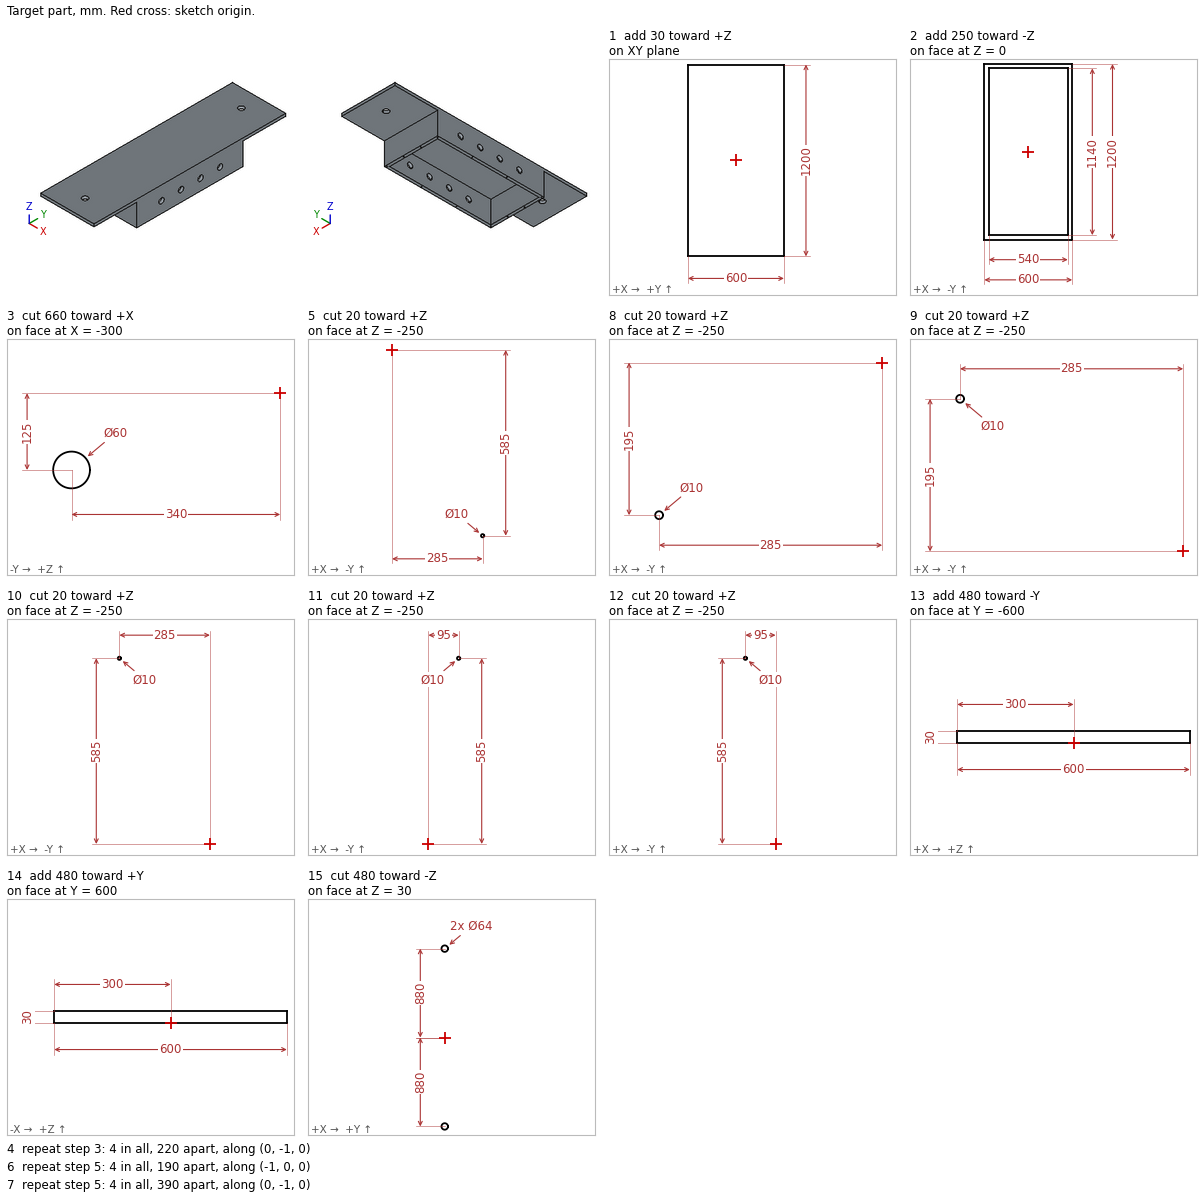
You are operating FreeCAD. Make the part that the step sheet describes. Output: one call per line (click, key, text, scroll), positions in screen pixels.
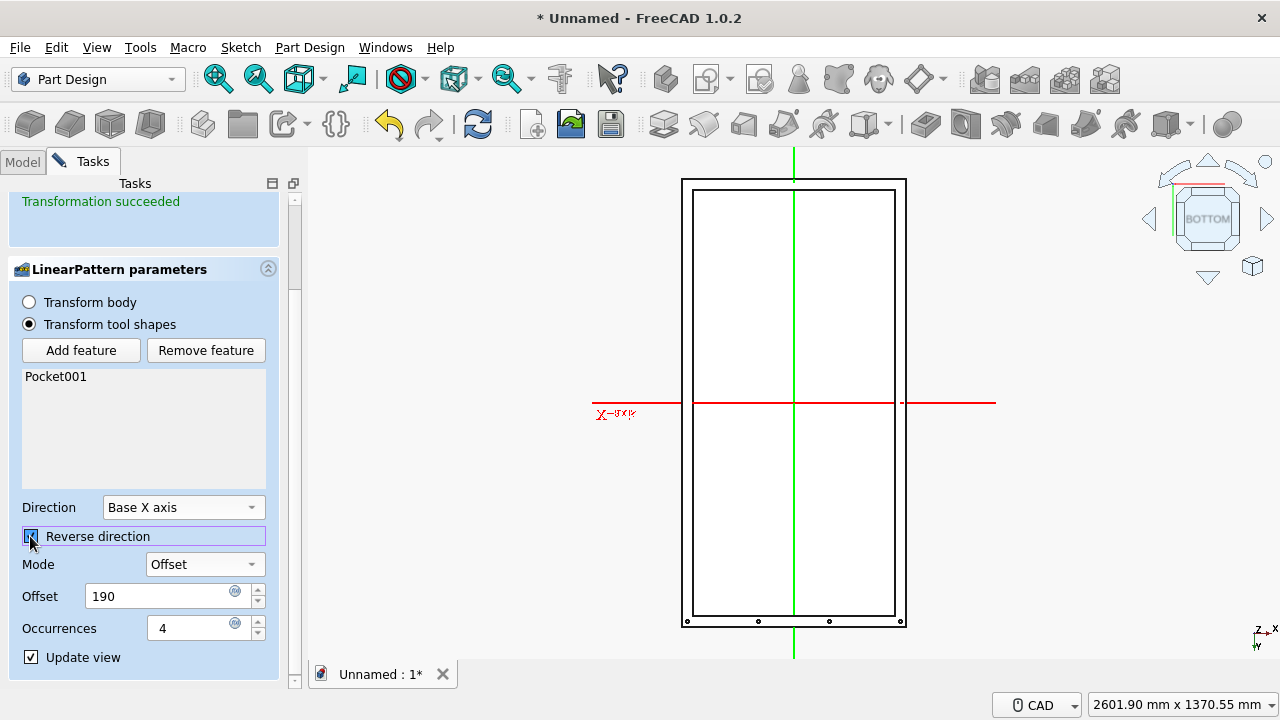
scroll(295, 440, up, 3)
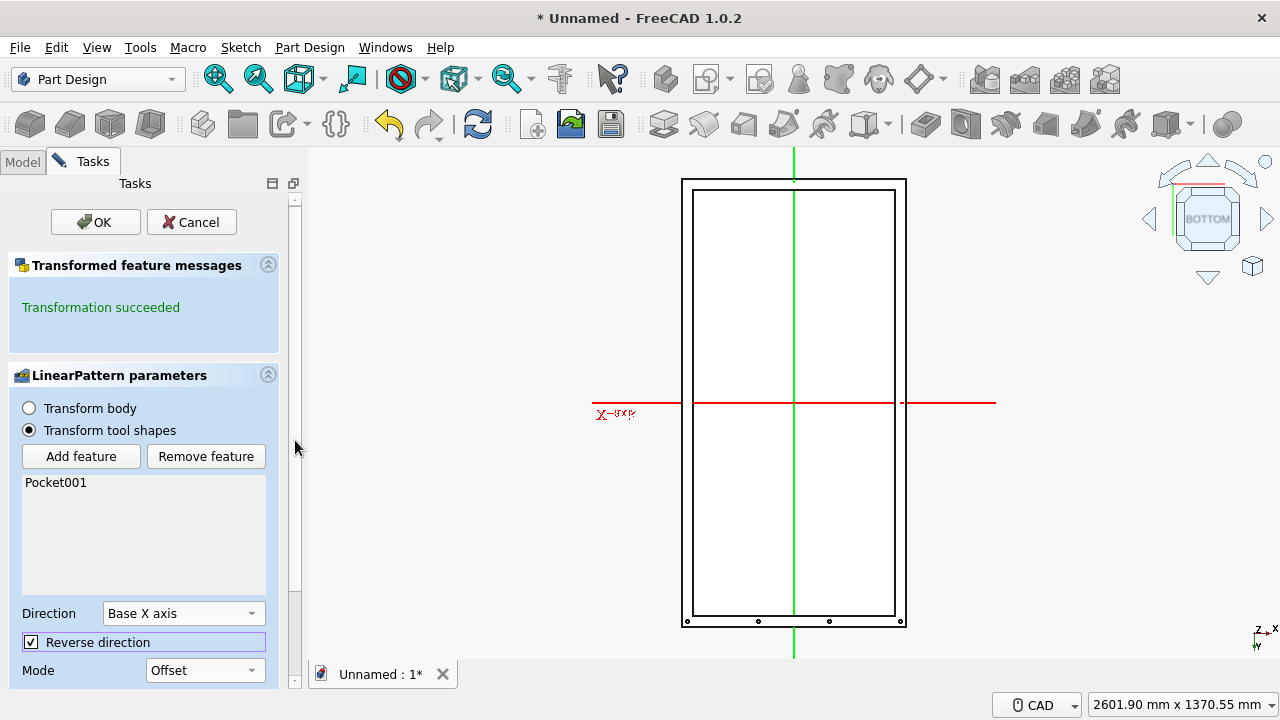
click(96, 222)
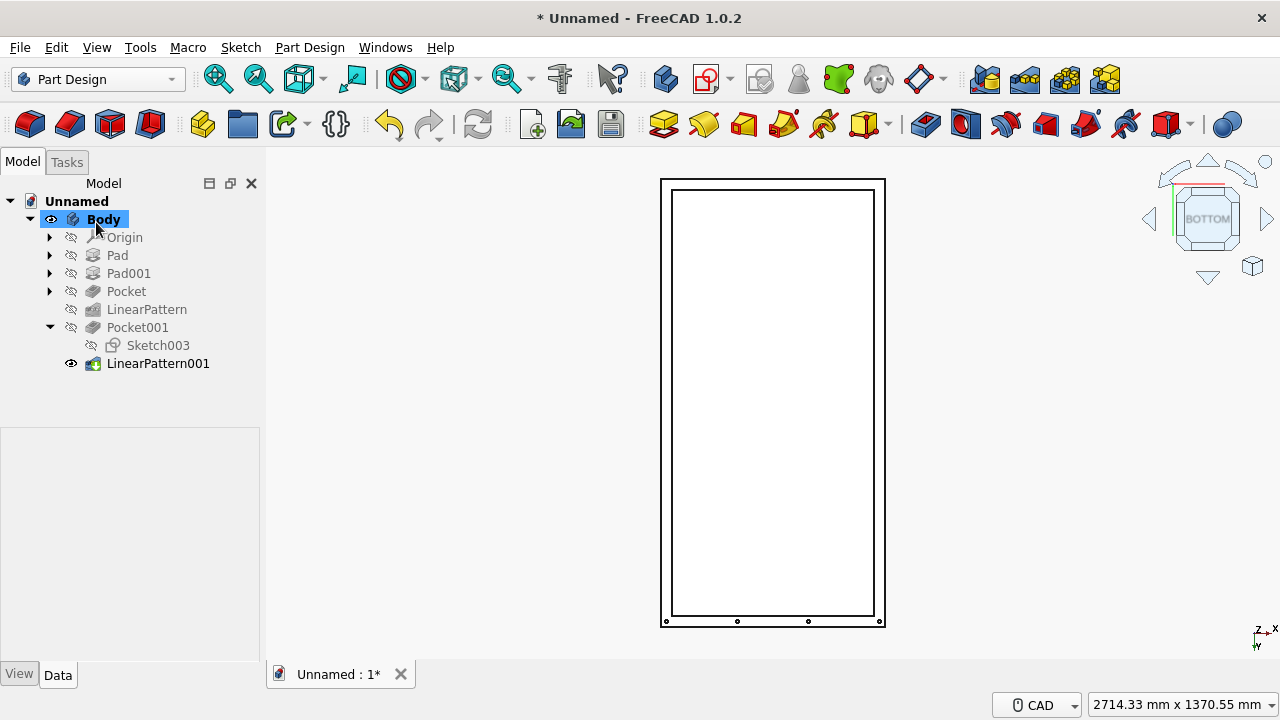
click(116, 327)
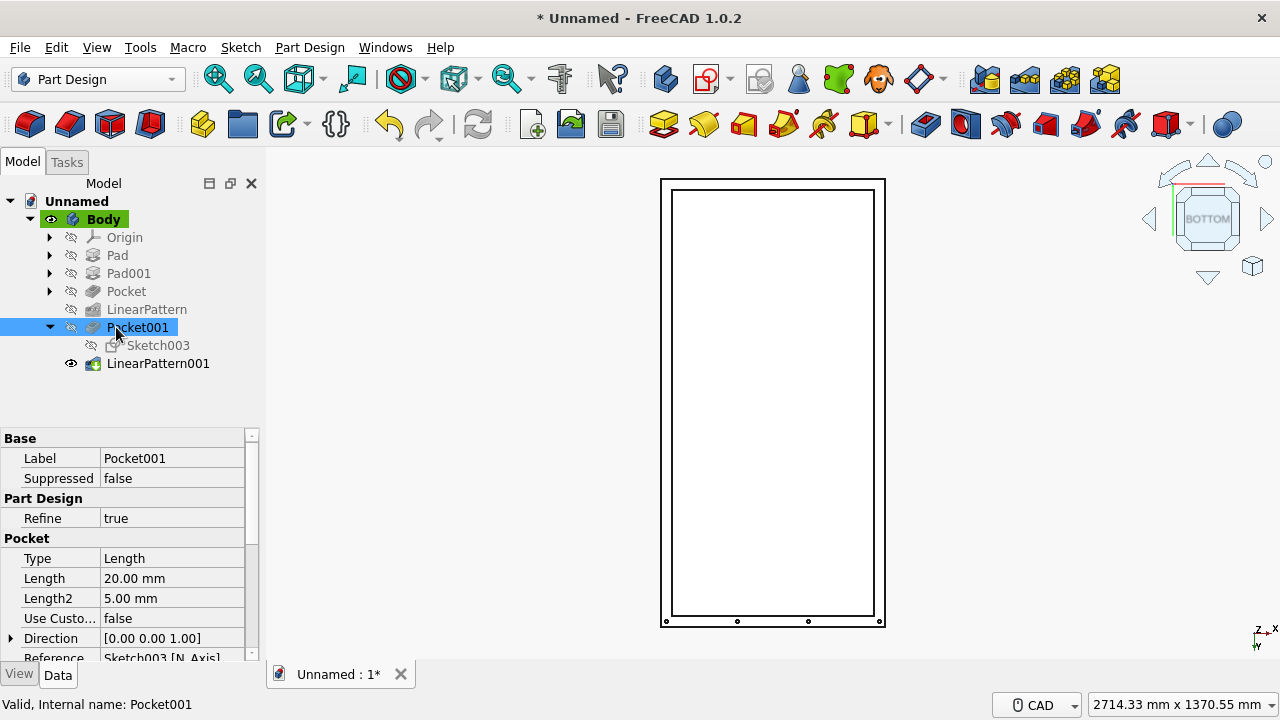
click(1026, 80)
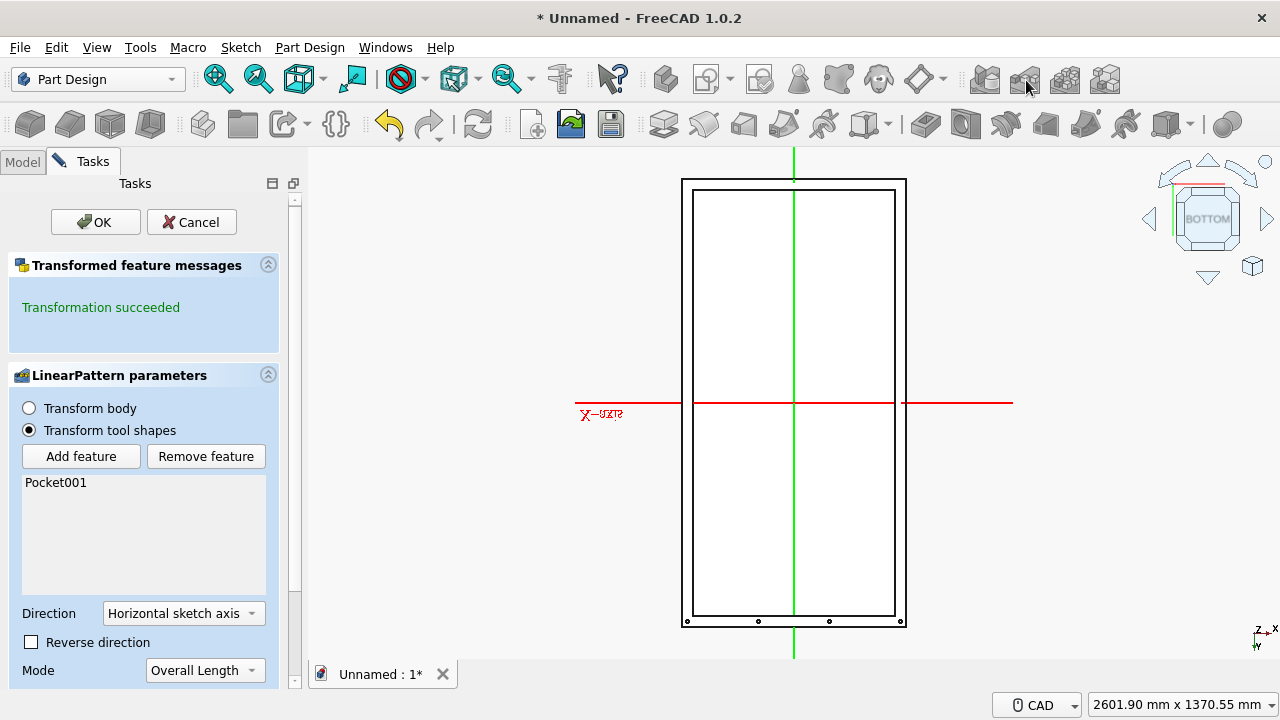
click(184, 614)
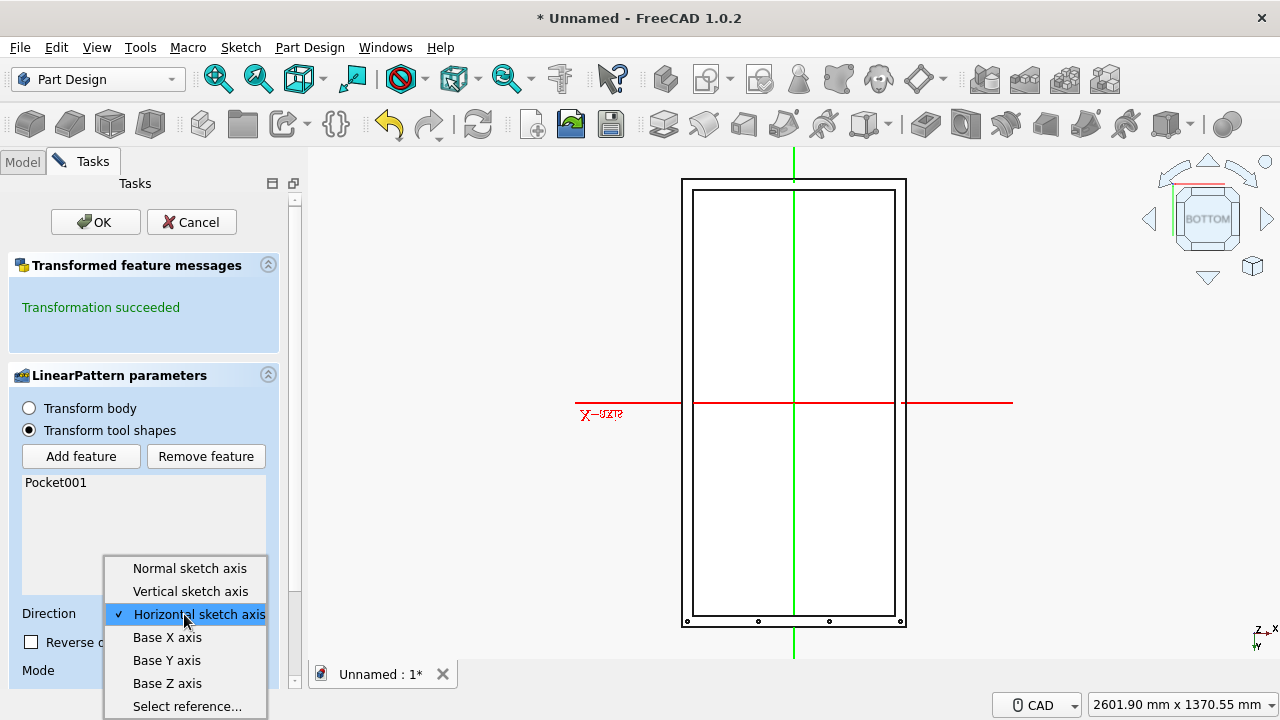
click(184, 660)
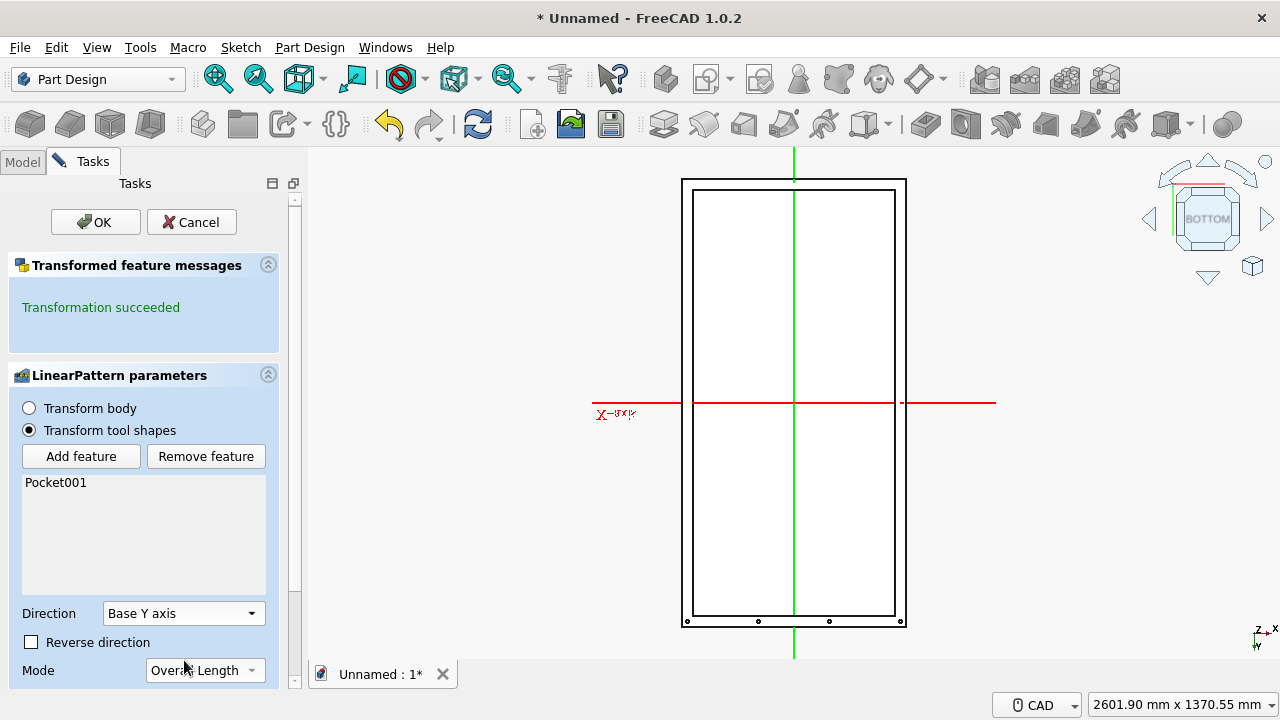
click(206, 670)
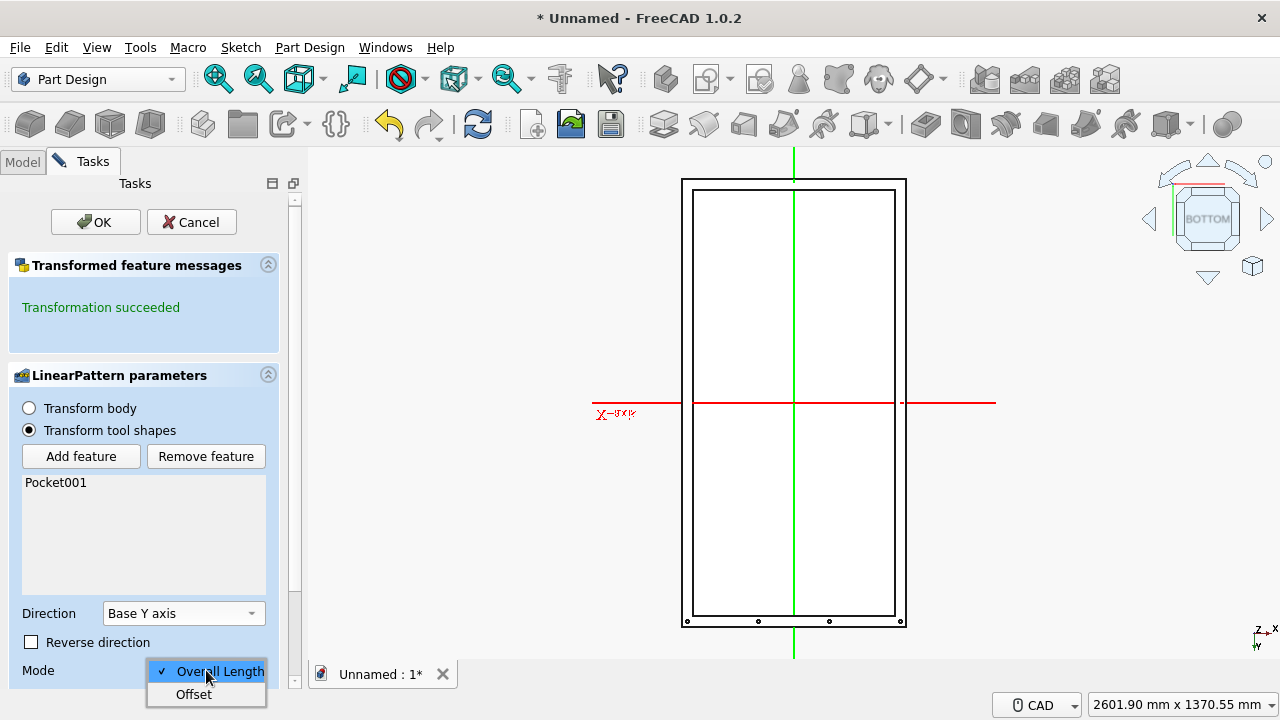
click(206, 694)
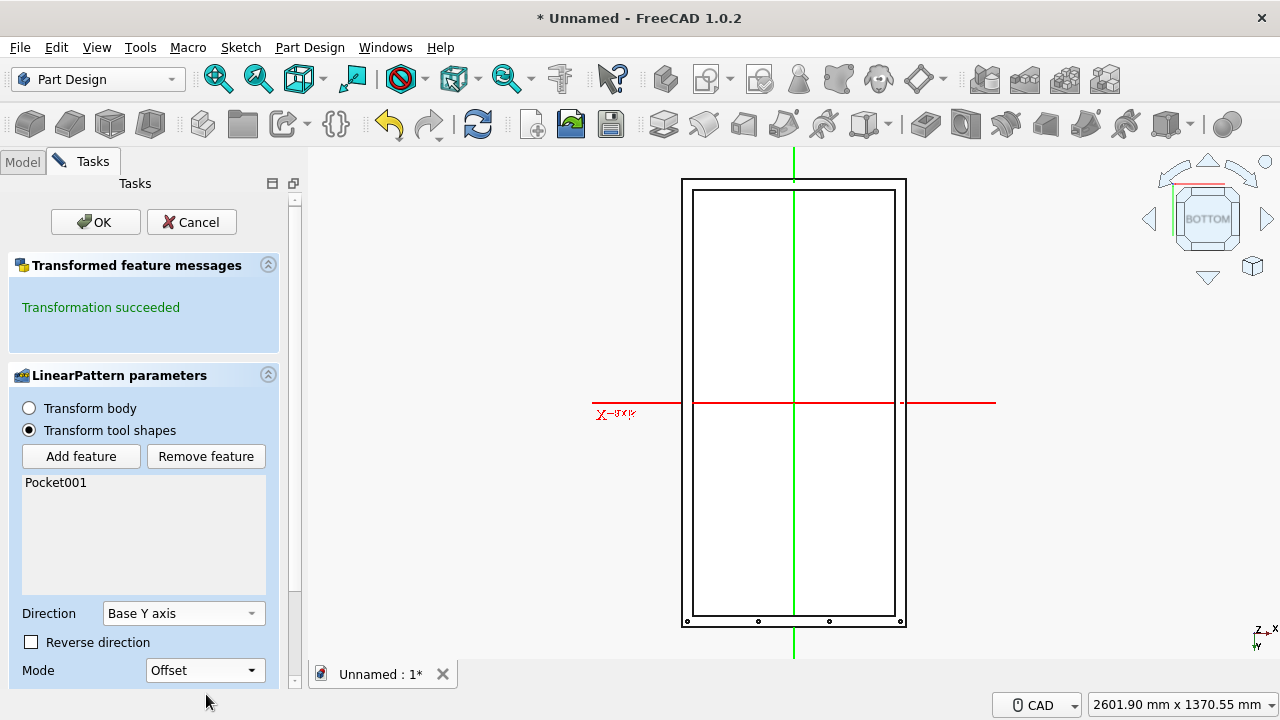
scroll(295, 440, down, 2)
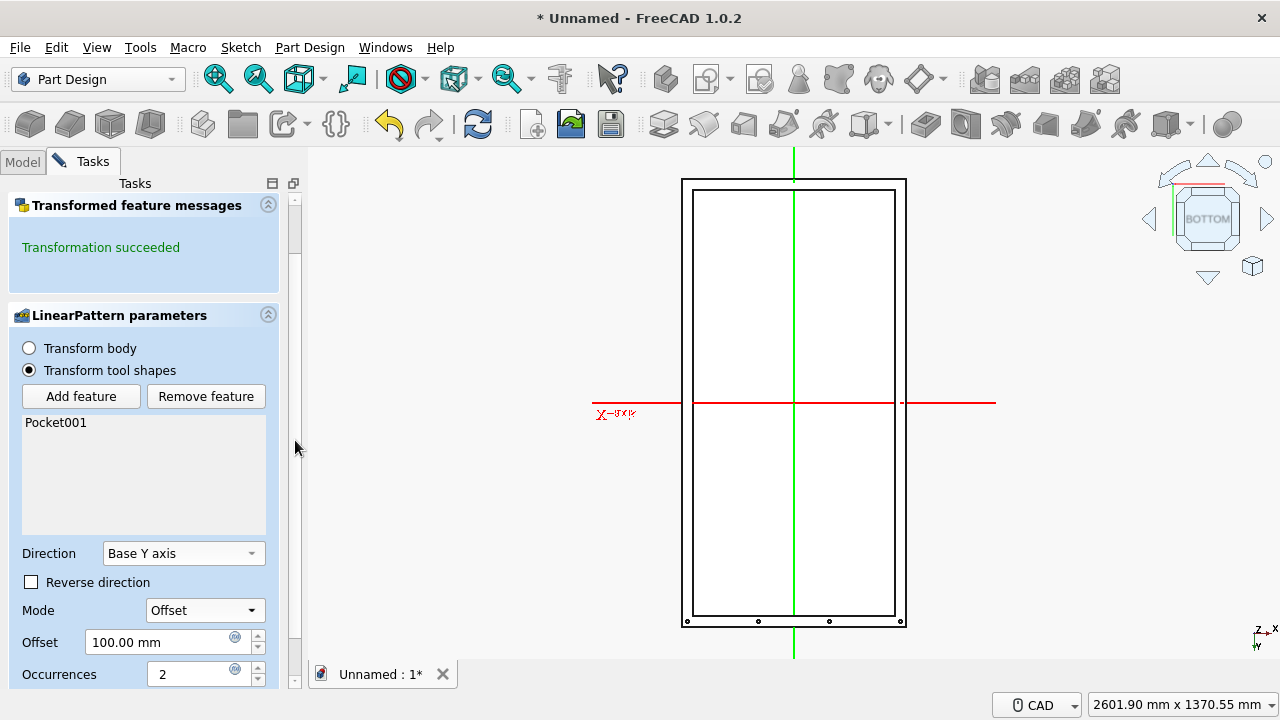
triple_click(168, 596)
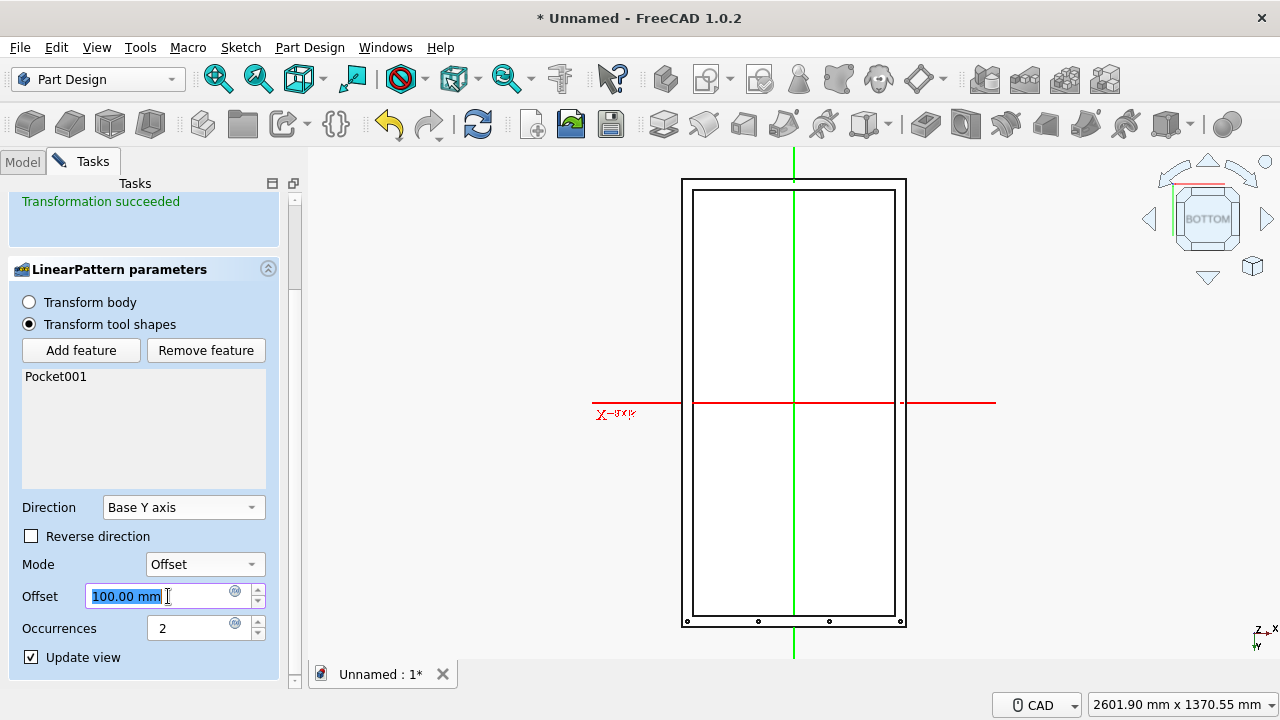
text(390)
key(Tab)